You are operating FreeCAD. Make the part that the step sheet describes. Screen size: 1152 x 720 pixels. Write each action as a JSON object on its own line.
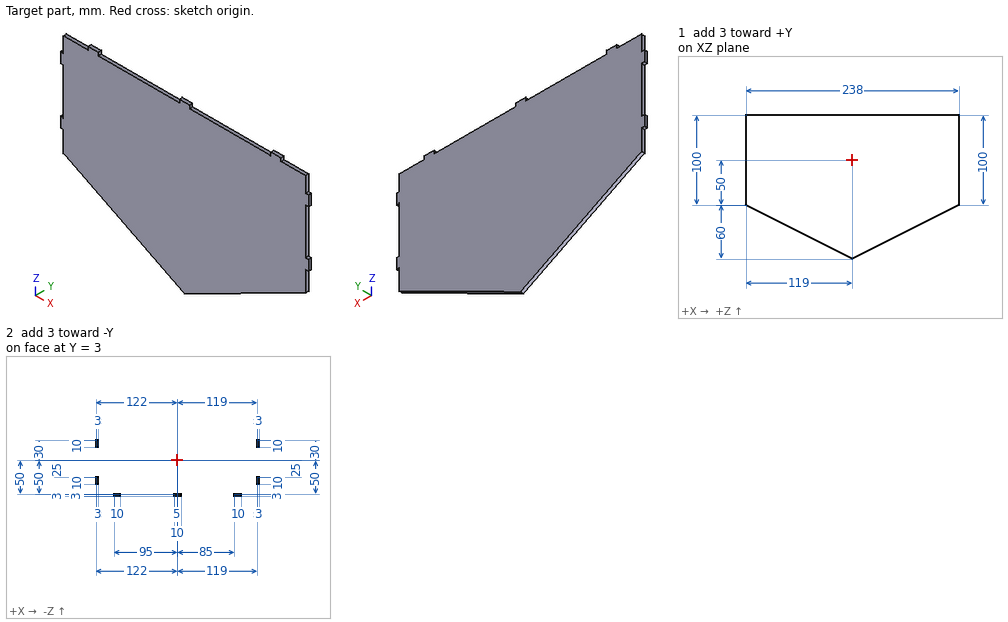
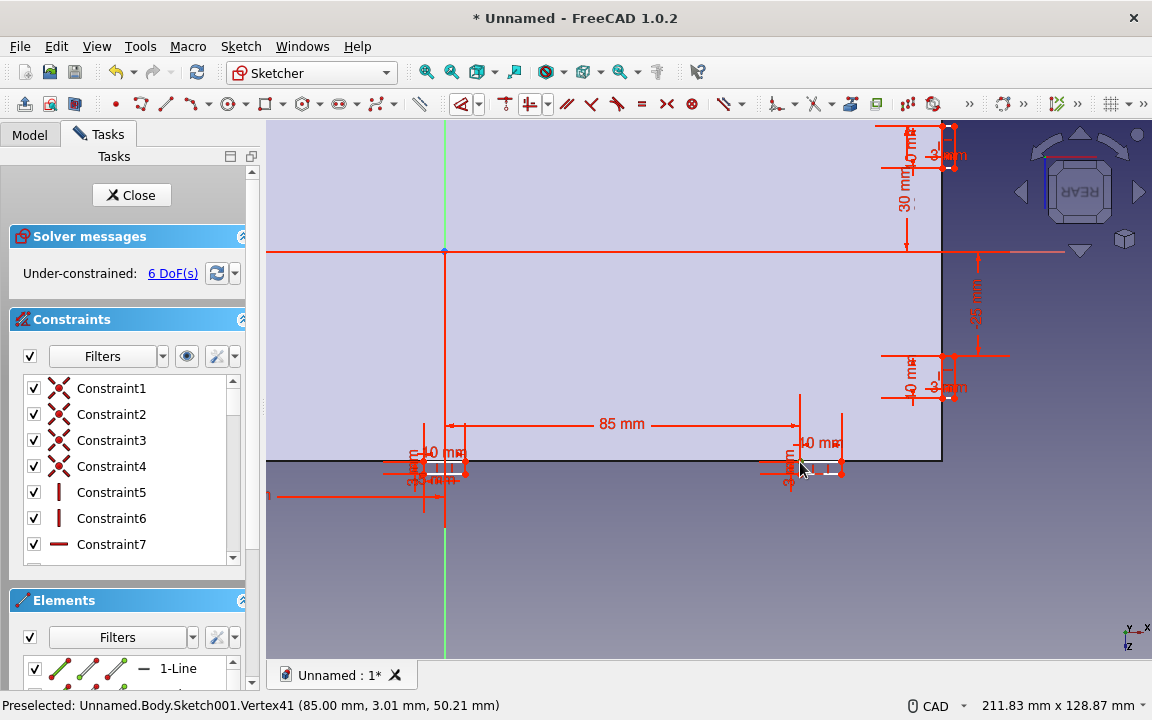
{"action": "key", "text": "i"}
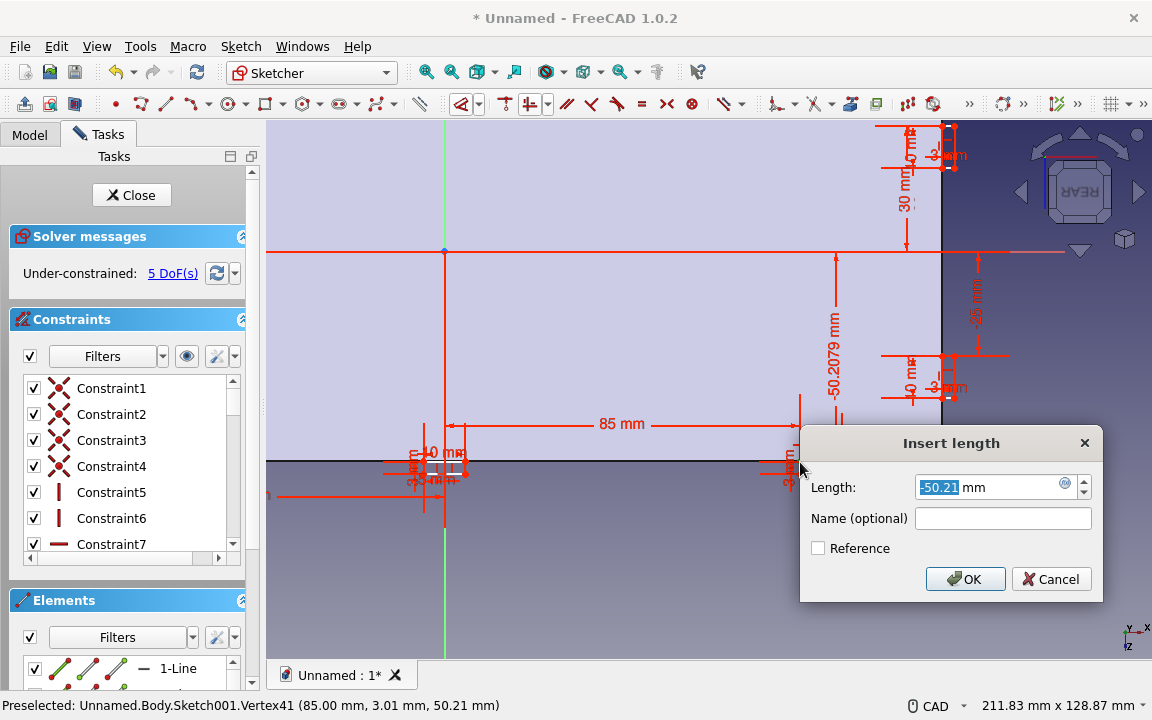
{"action": "type", "text": "-50"}
{"action": "key", "text": "Return"}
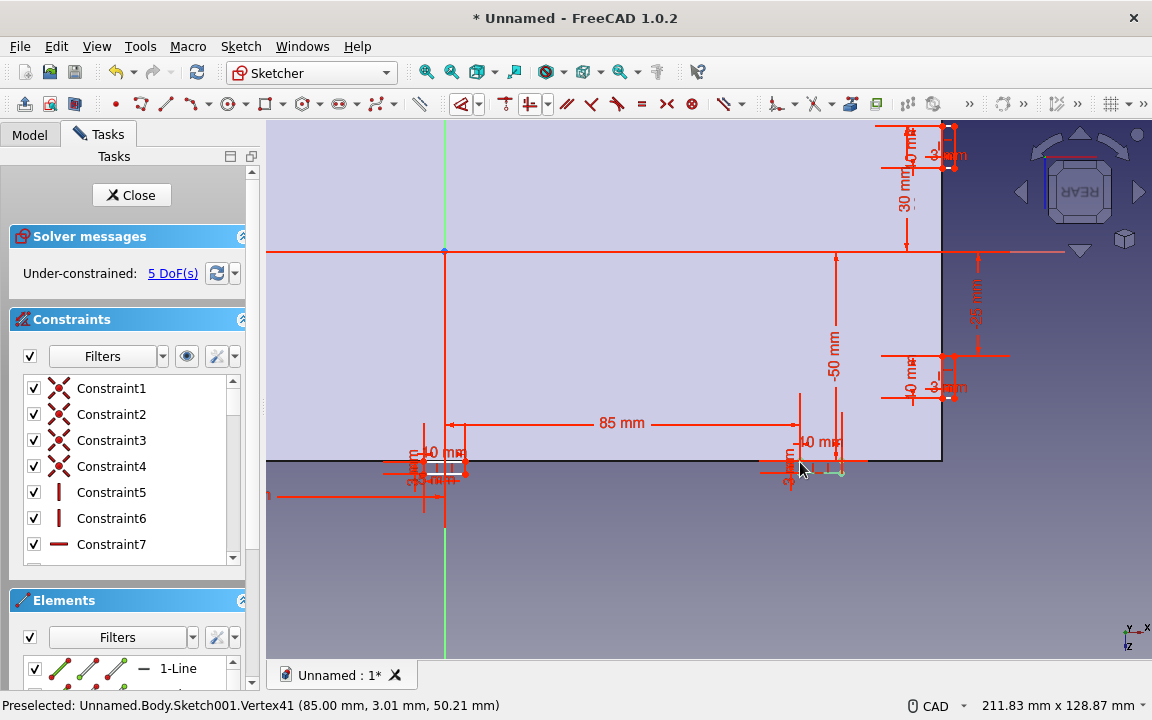
{"action": "left_click", "coordinate": [424, 462]}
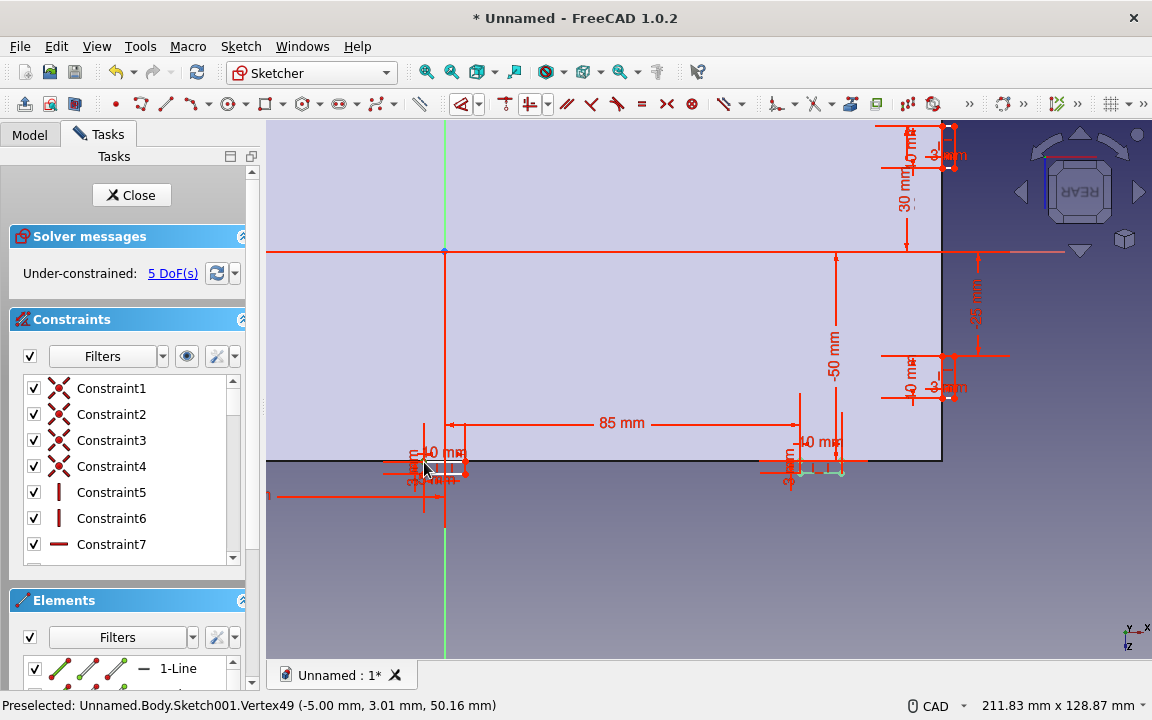
{"action": "key", "text": "i"}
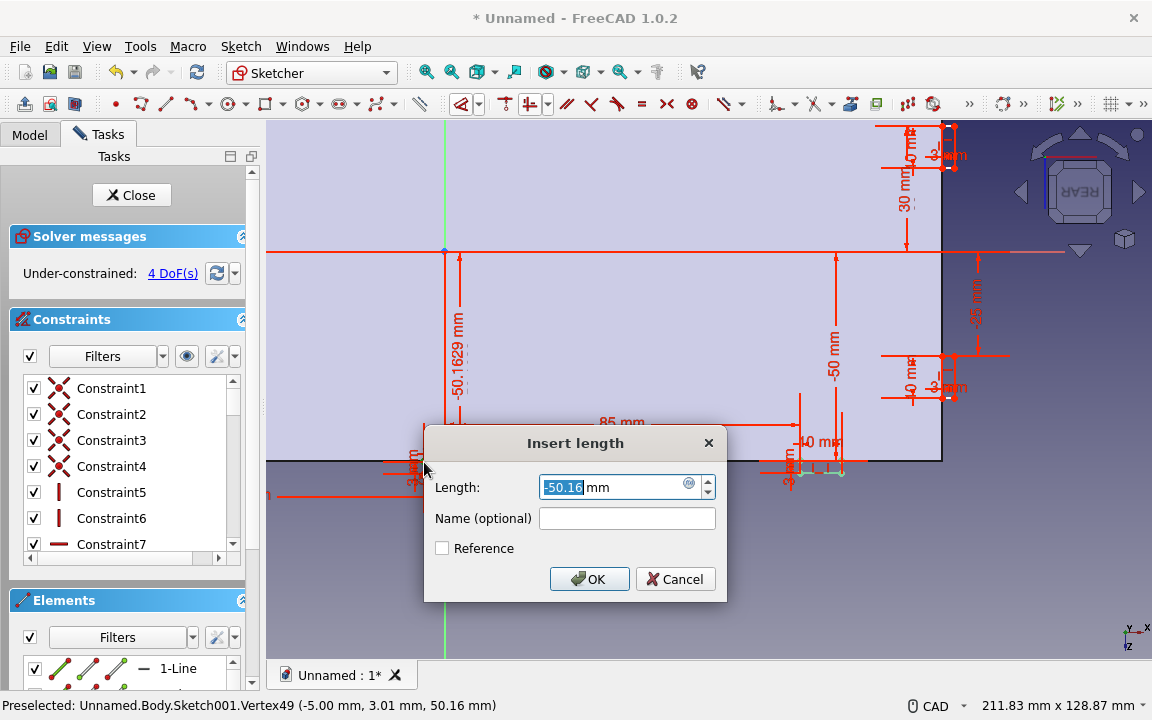
{"action": "type", "text": "-50"}
{"action": "key", "text": "Return"}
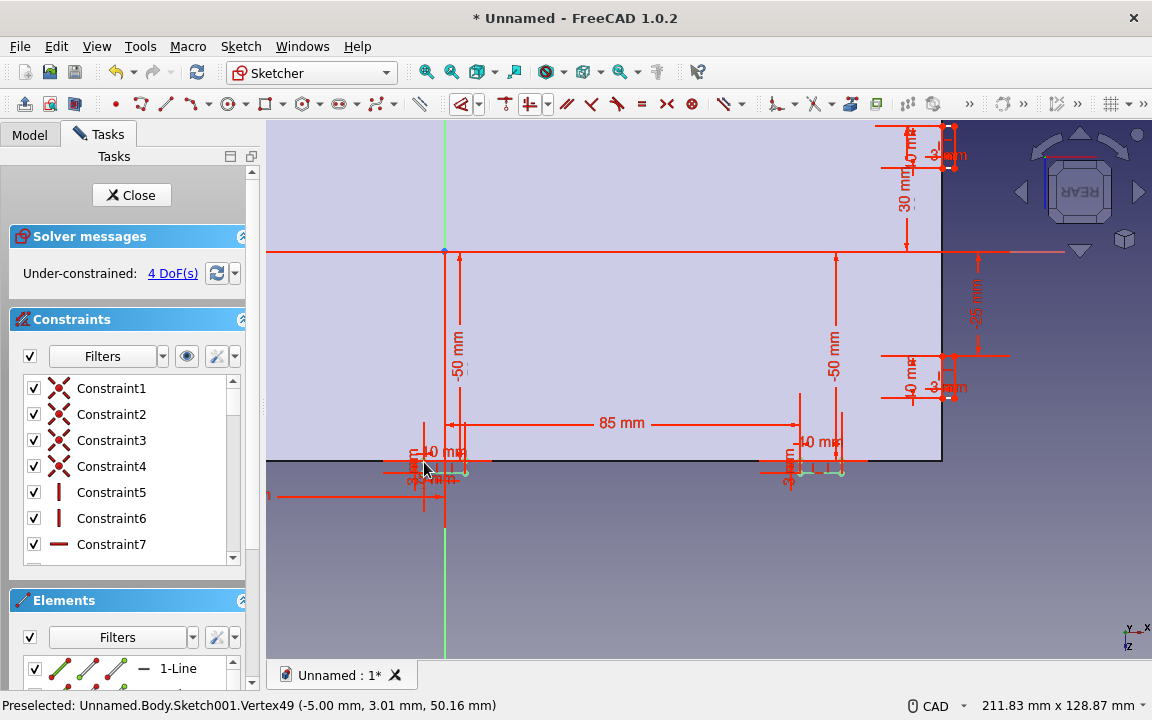
{"action": "scroll", "coordinate": [800, 463], "scroll_direction": "down", "scroll_amount": 4}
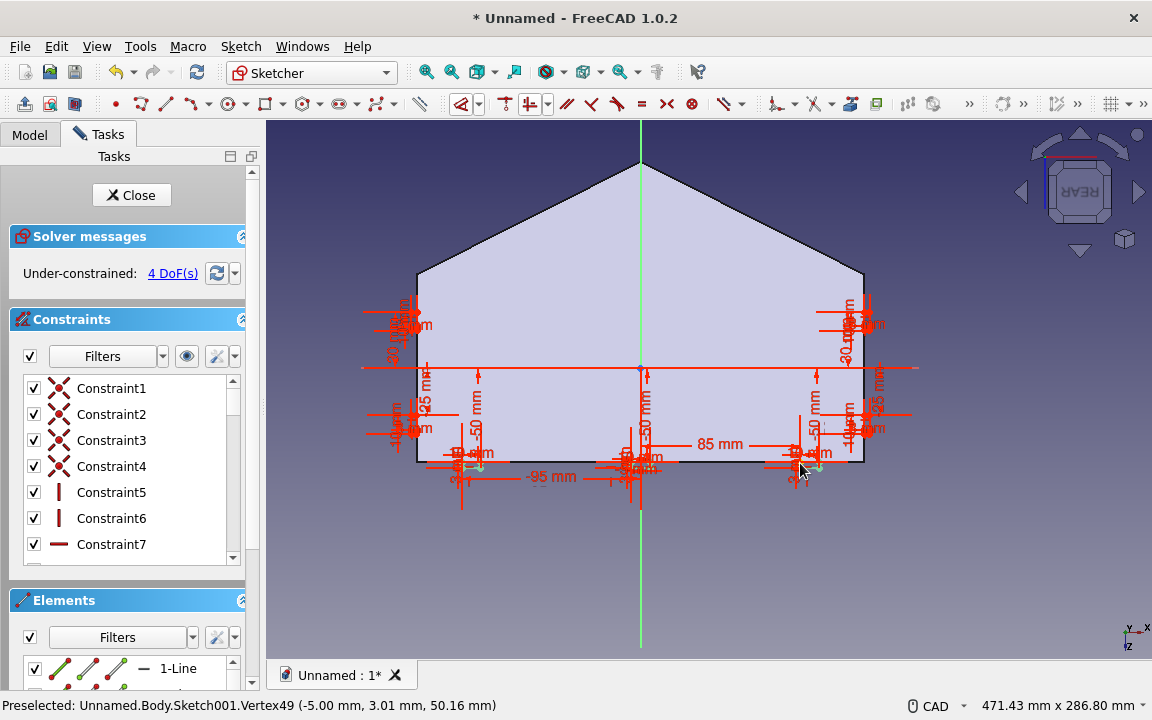
{"action": "scroll", "coordinate": [864, 312], "scroll_direction": "up", "scroll_amount": 4}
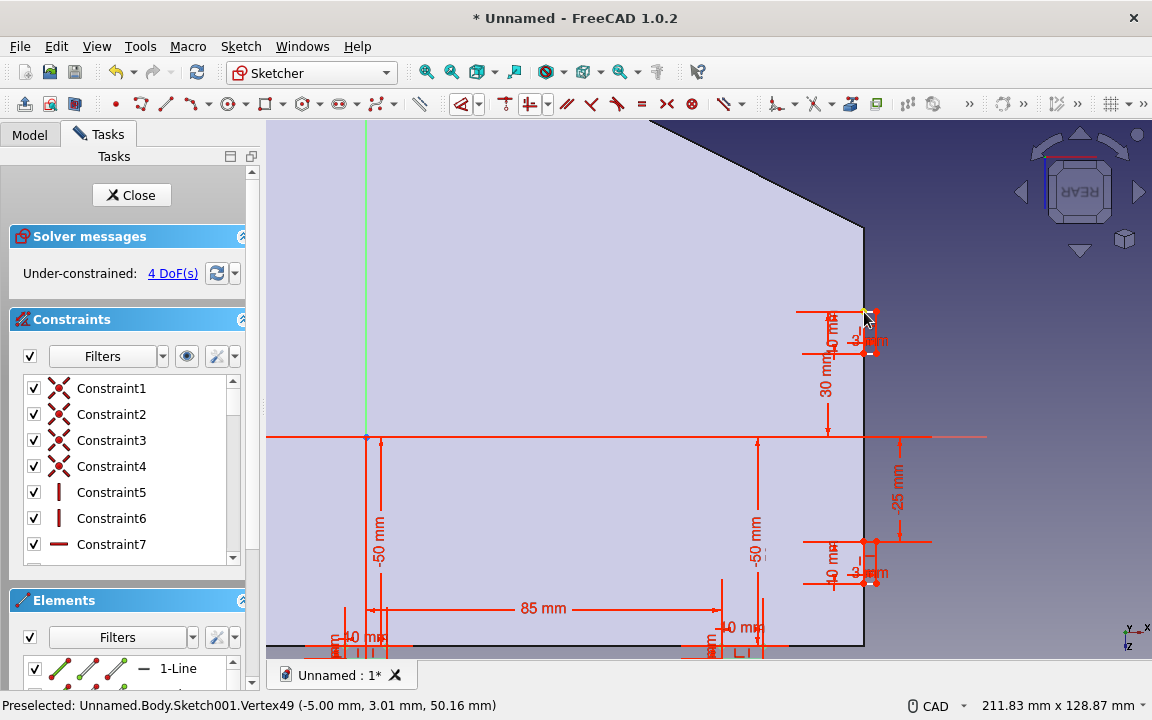
{"action": "left_click", "coordinate": [864, 312]}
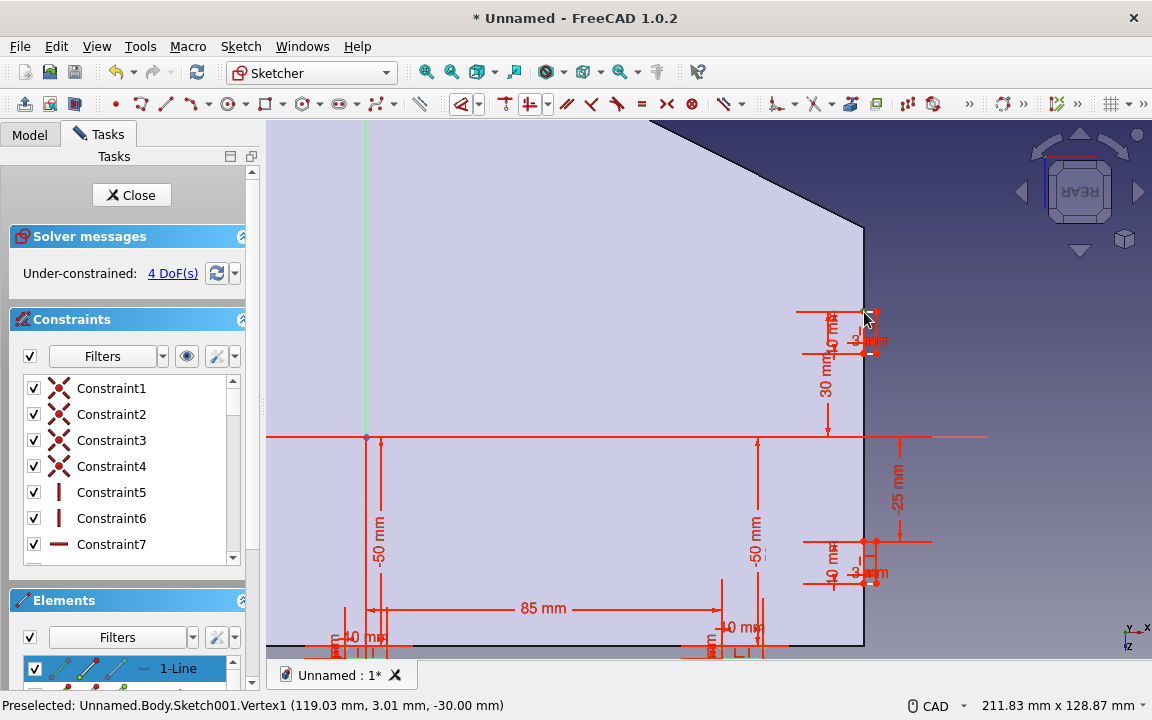
{"action": "key", "text": "l"}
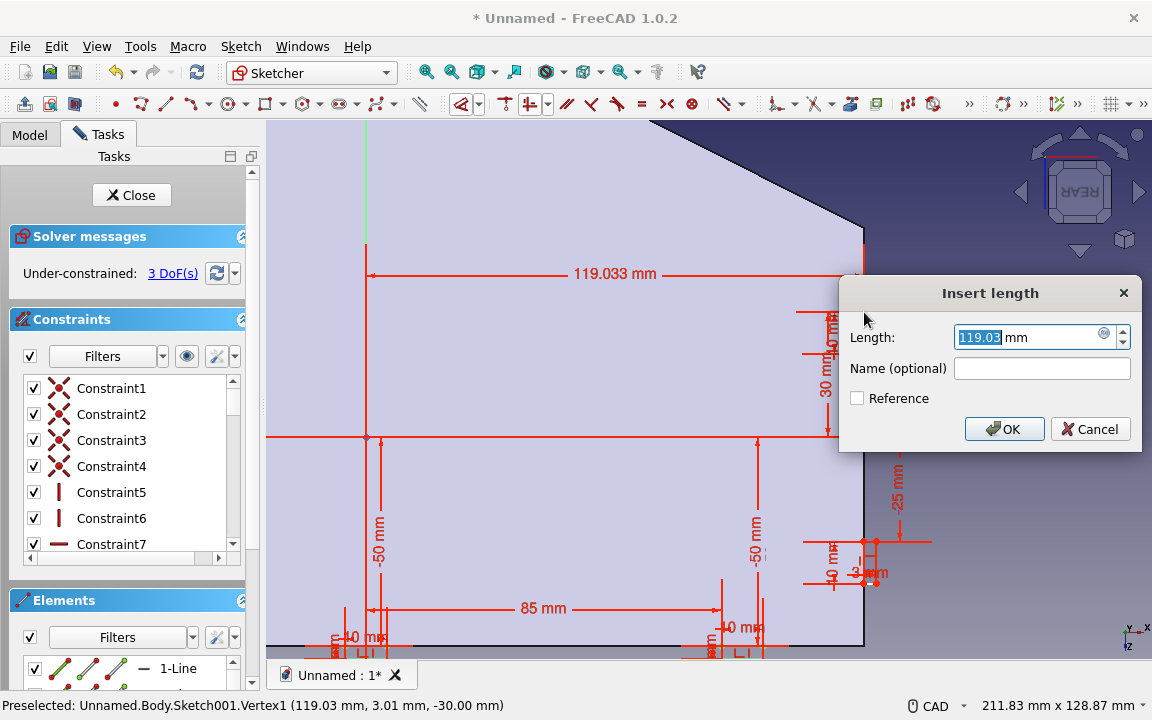
{"action": "type", "text": "119"}
{"action": "key", "text": "Return"}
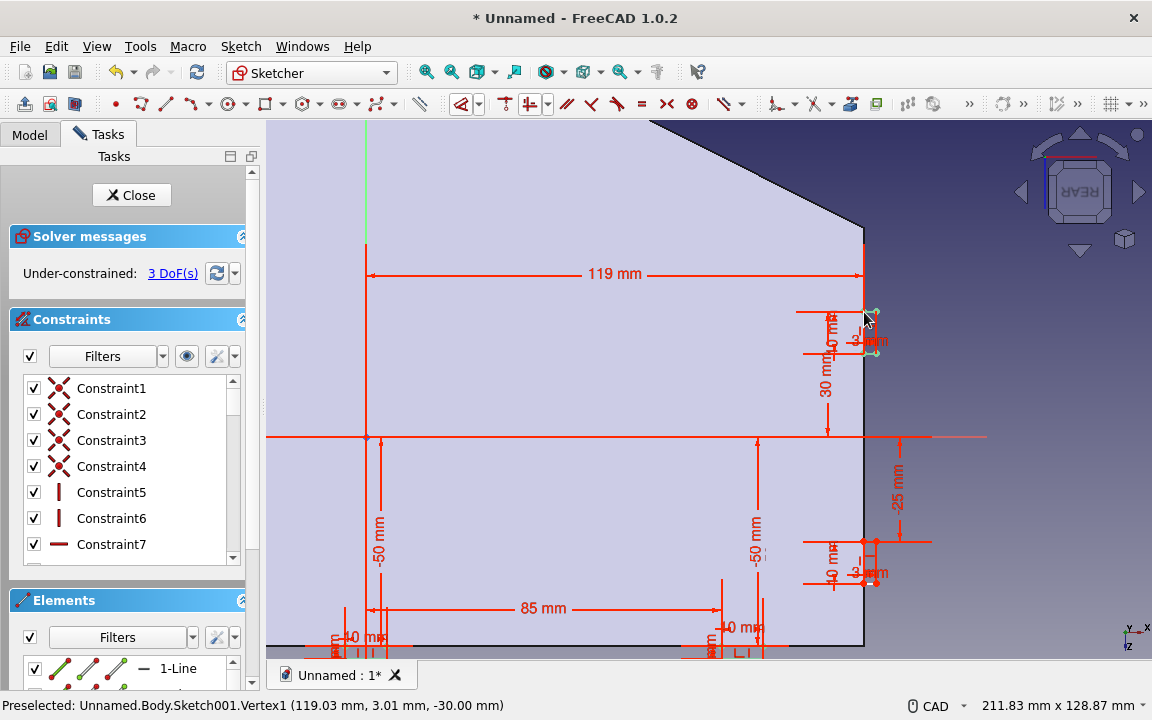
{"action": "left_click", "coordinate": [864, 542]}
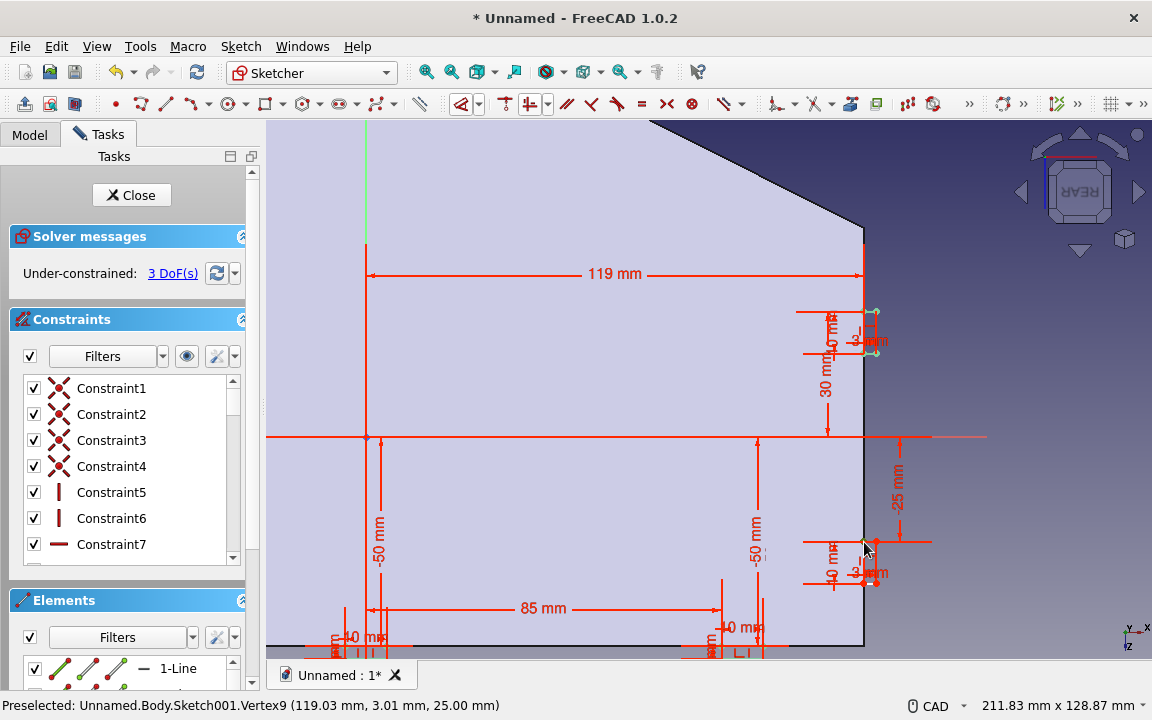
{"action": "key", "text": "l"}